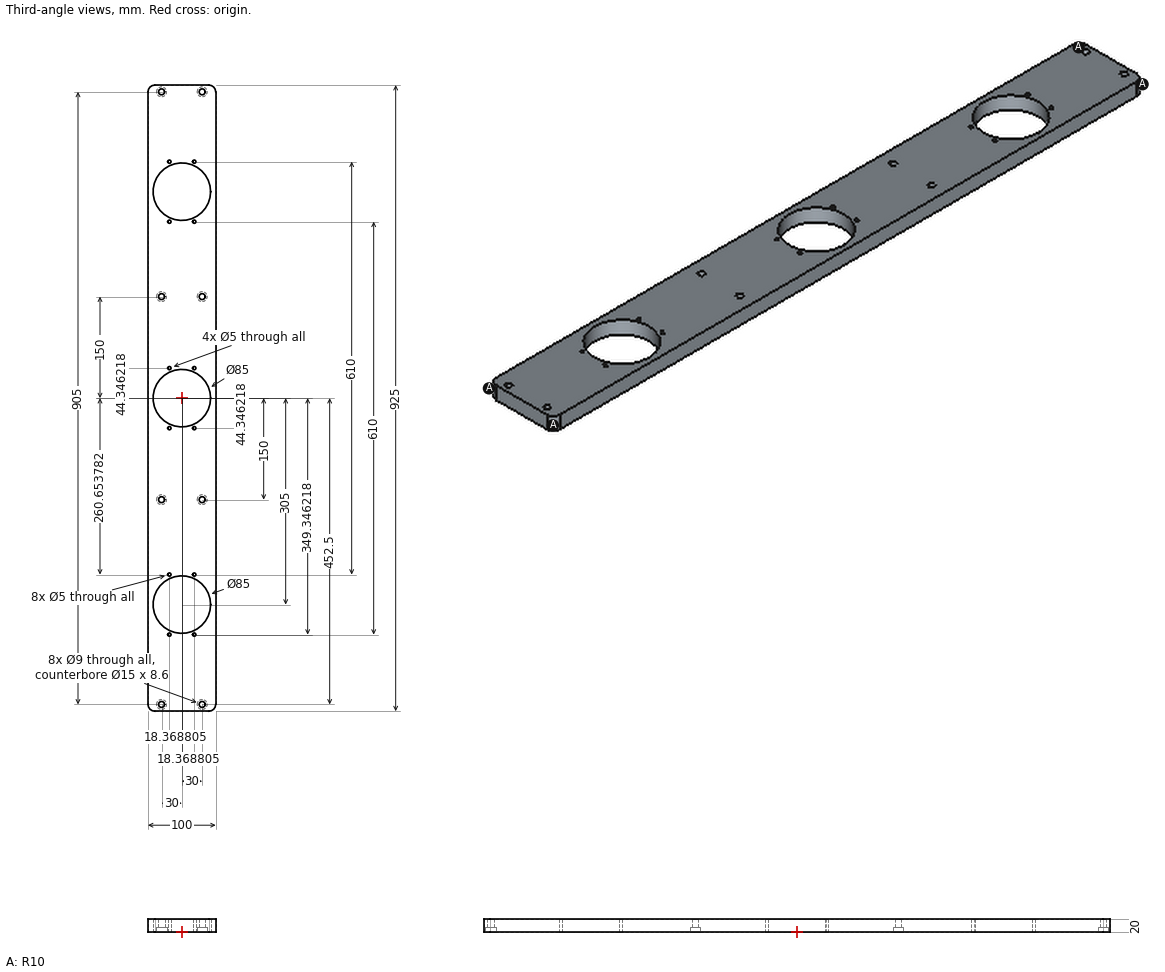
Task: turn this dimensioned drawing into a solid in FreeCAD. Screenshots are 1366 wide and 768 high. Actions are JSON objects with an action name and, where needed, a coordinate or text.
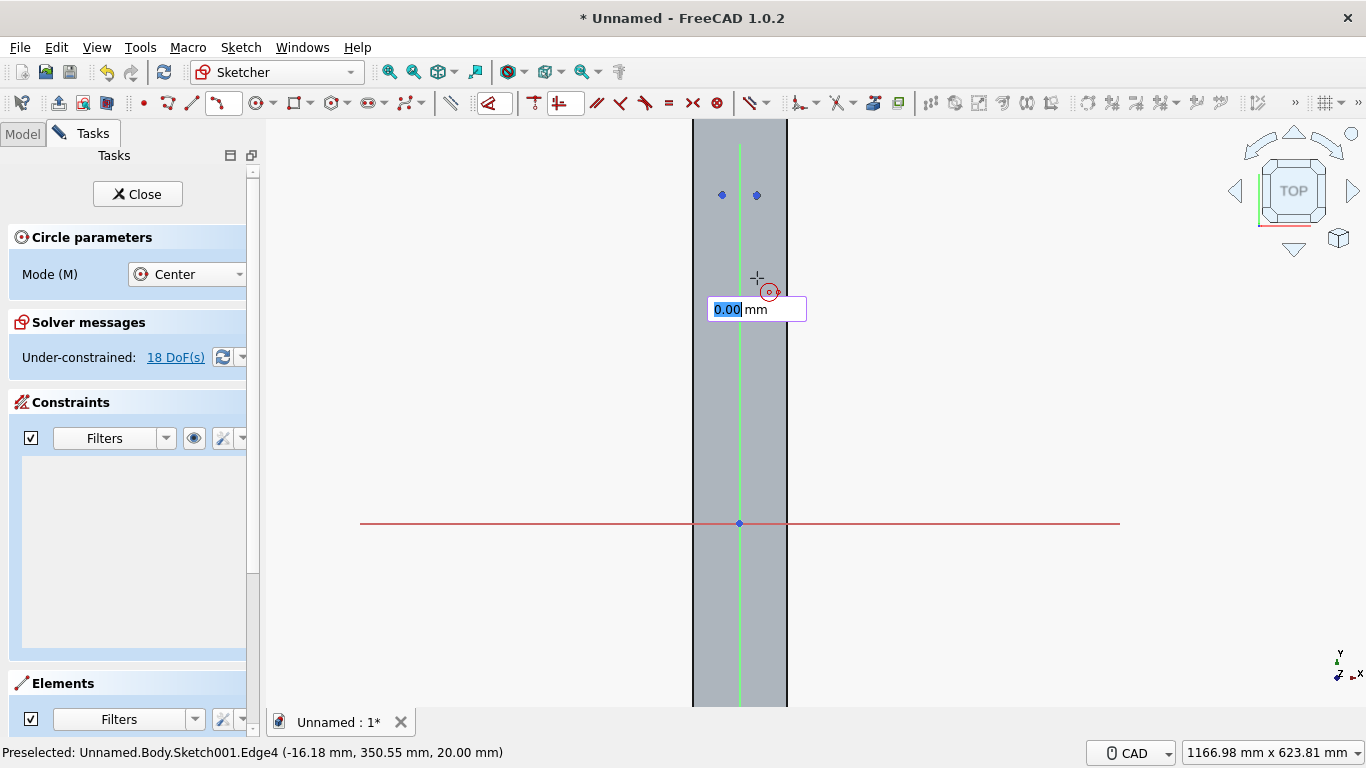
{"action": "scroll", "coordinate": [759, 277], "scroll_direction": "up", "scroll_amount": 10}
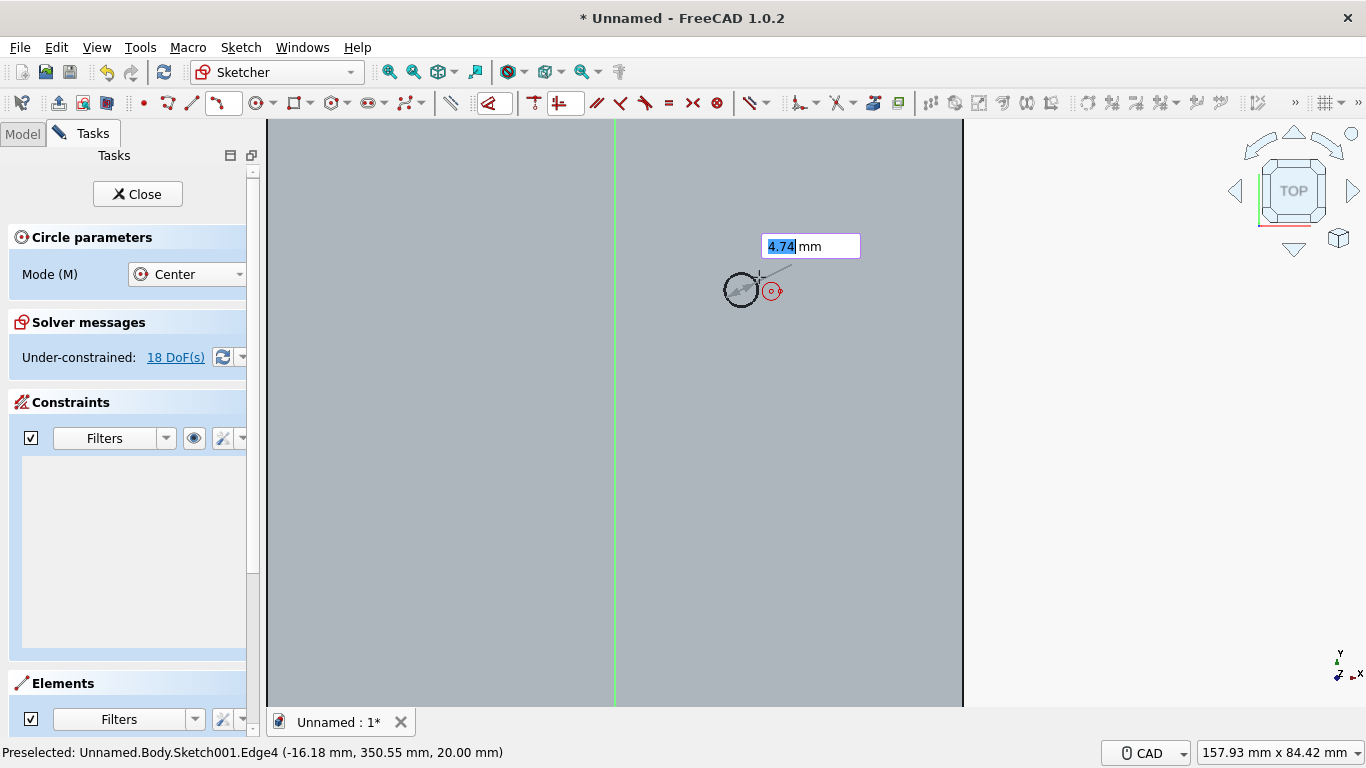
{"action": "left_click", "coordinate": [755, 272]}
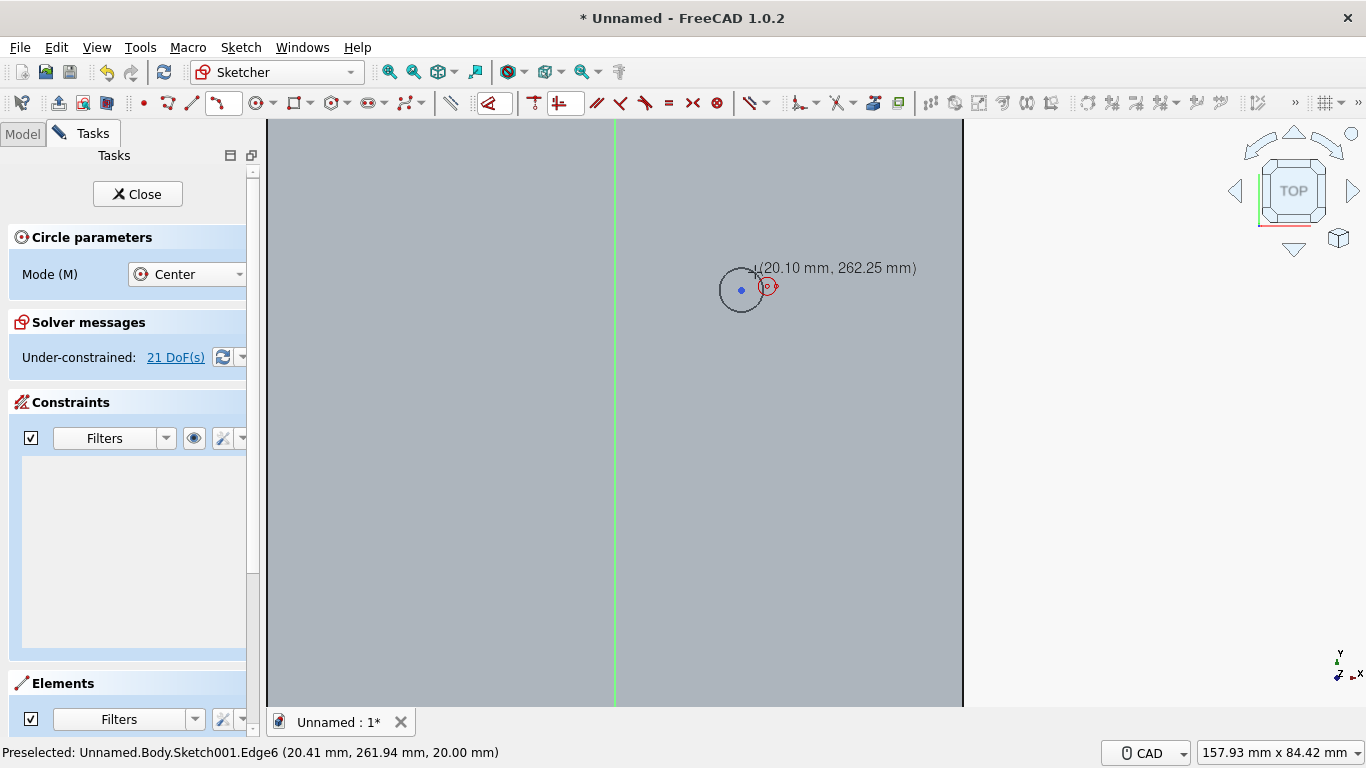
{"action": "scroll", "coordinate": [487, 284], "scroll_direction": "up", "scroll_amount": 2}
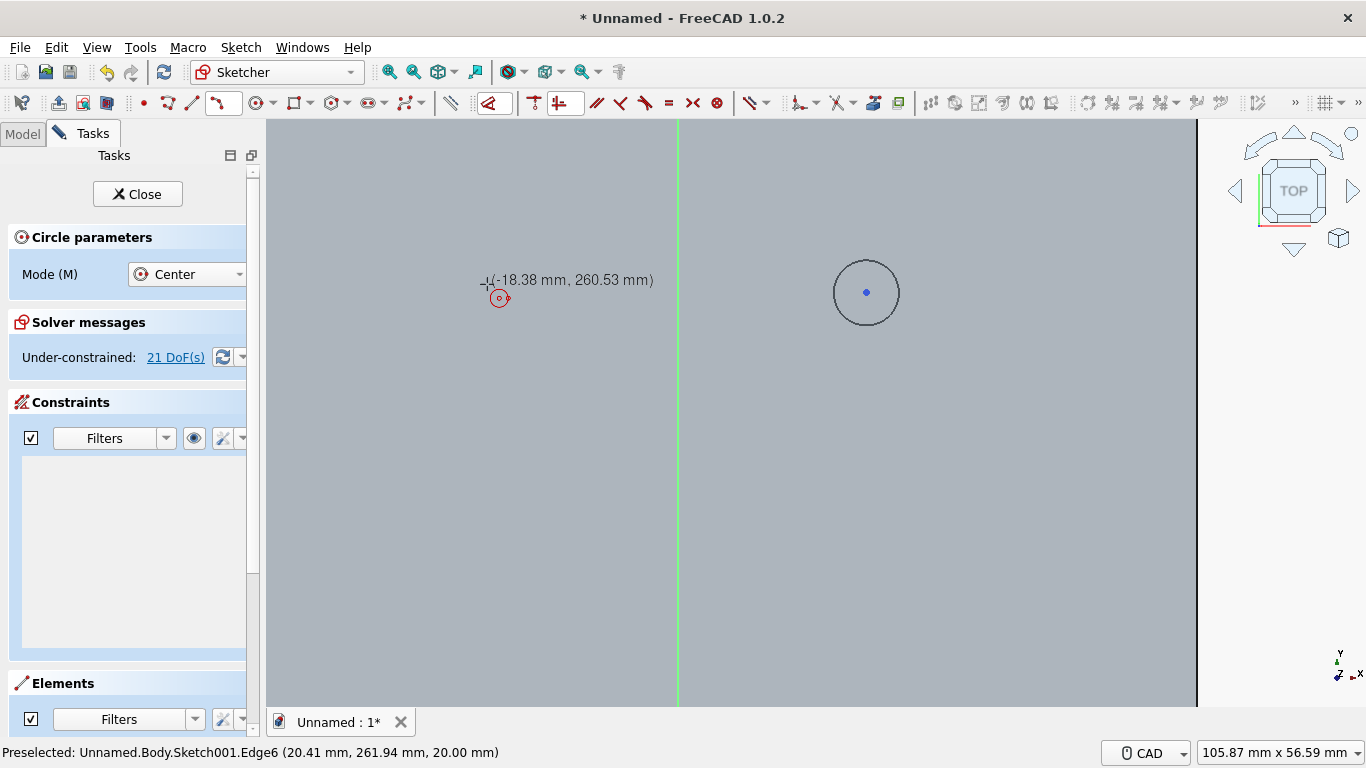
{"action": "scroll", "coordinate": [751, 278], "scroll_direction": "down", "scroll_amount": 15}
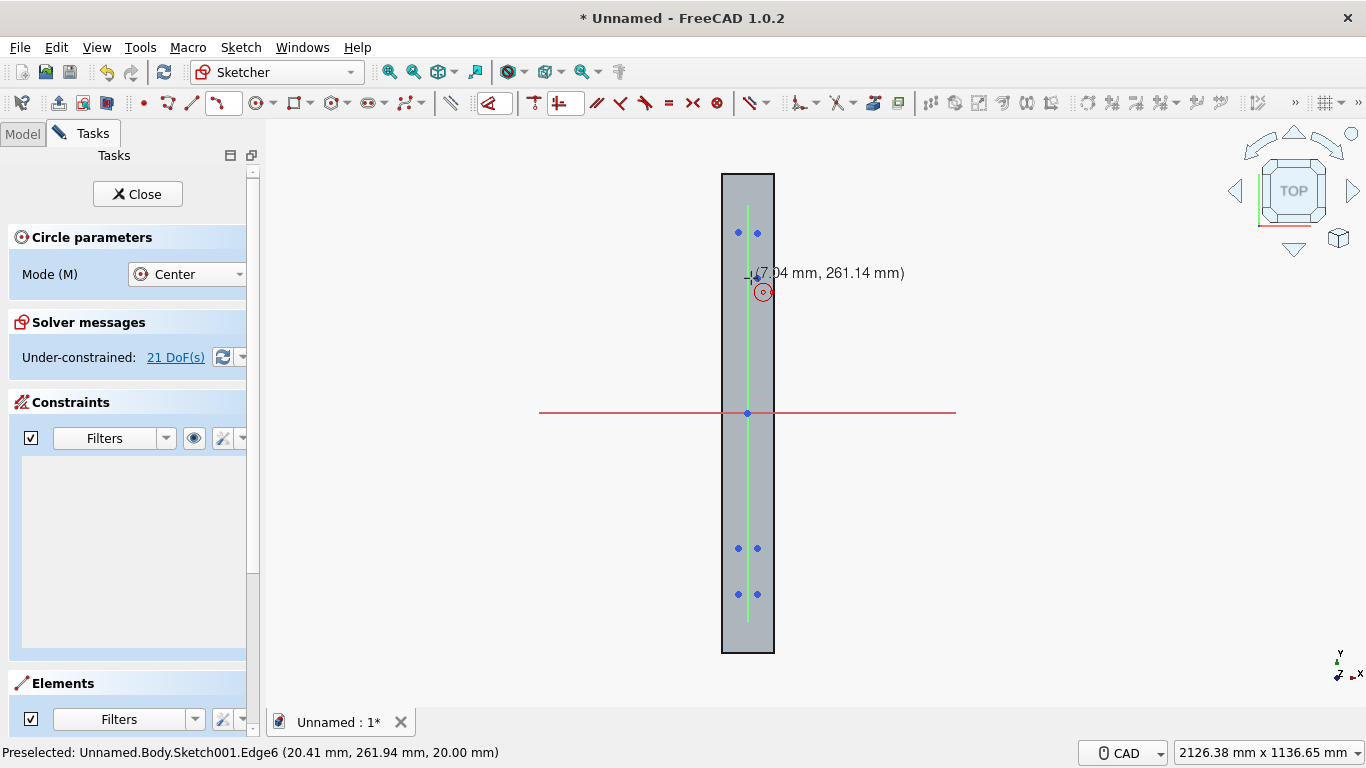
{"action": "scroll", "coordinate": [738, 279], "scroll_direction": "up", "scroll_amount": 3}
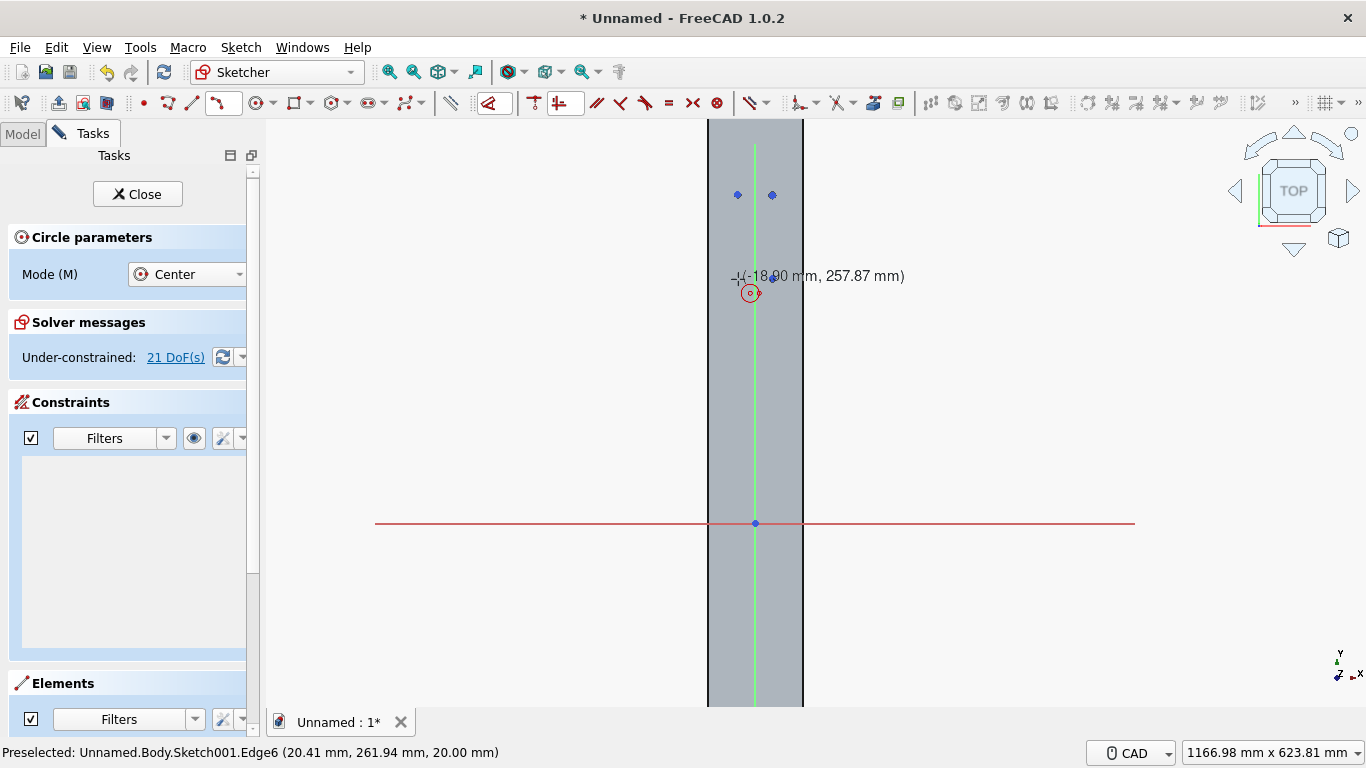
{"action": "left_click", "coordinate": [738, 278]}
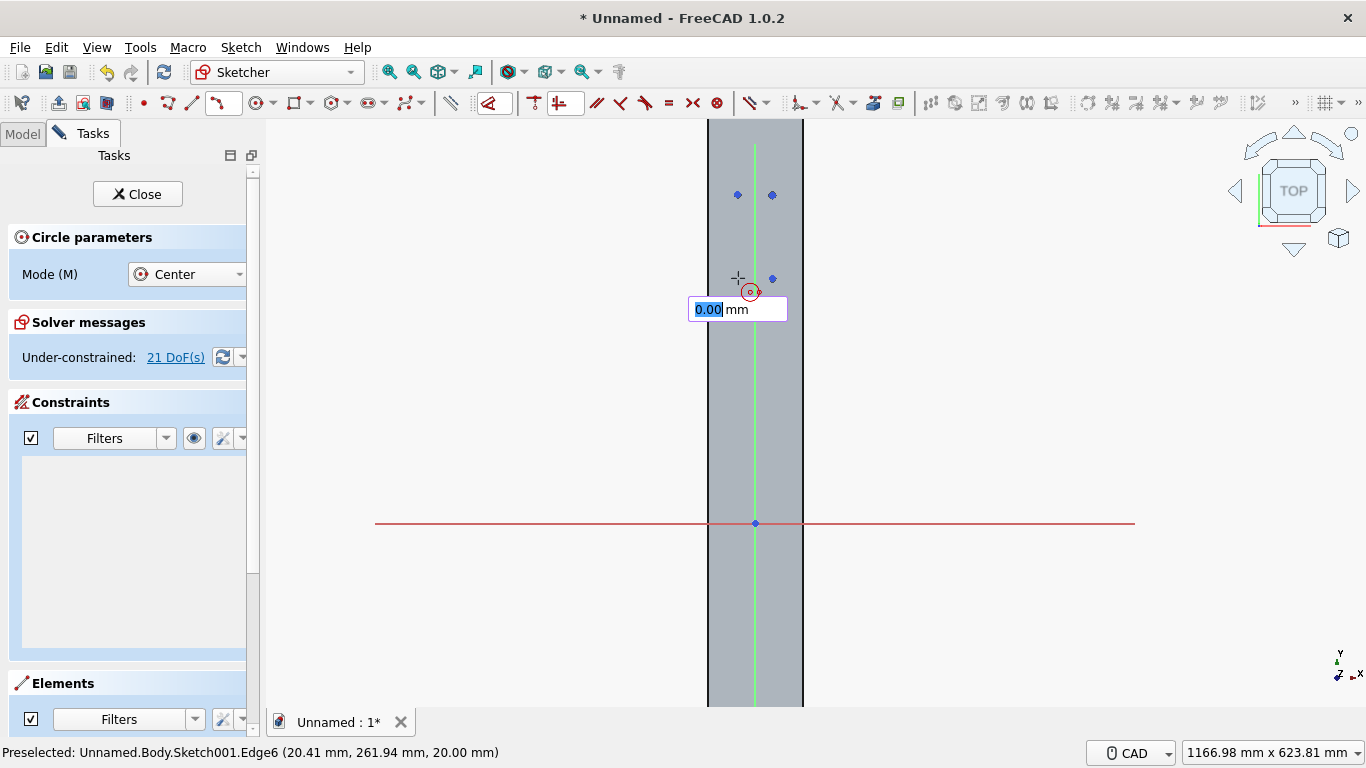
{"action": "scroll", "coordinate": [740, 276], "scroll_direction": "up", "scroll_amount": 10}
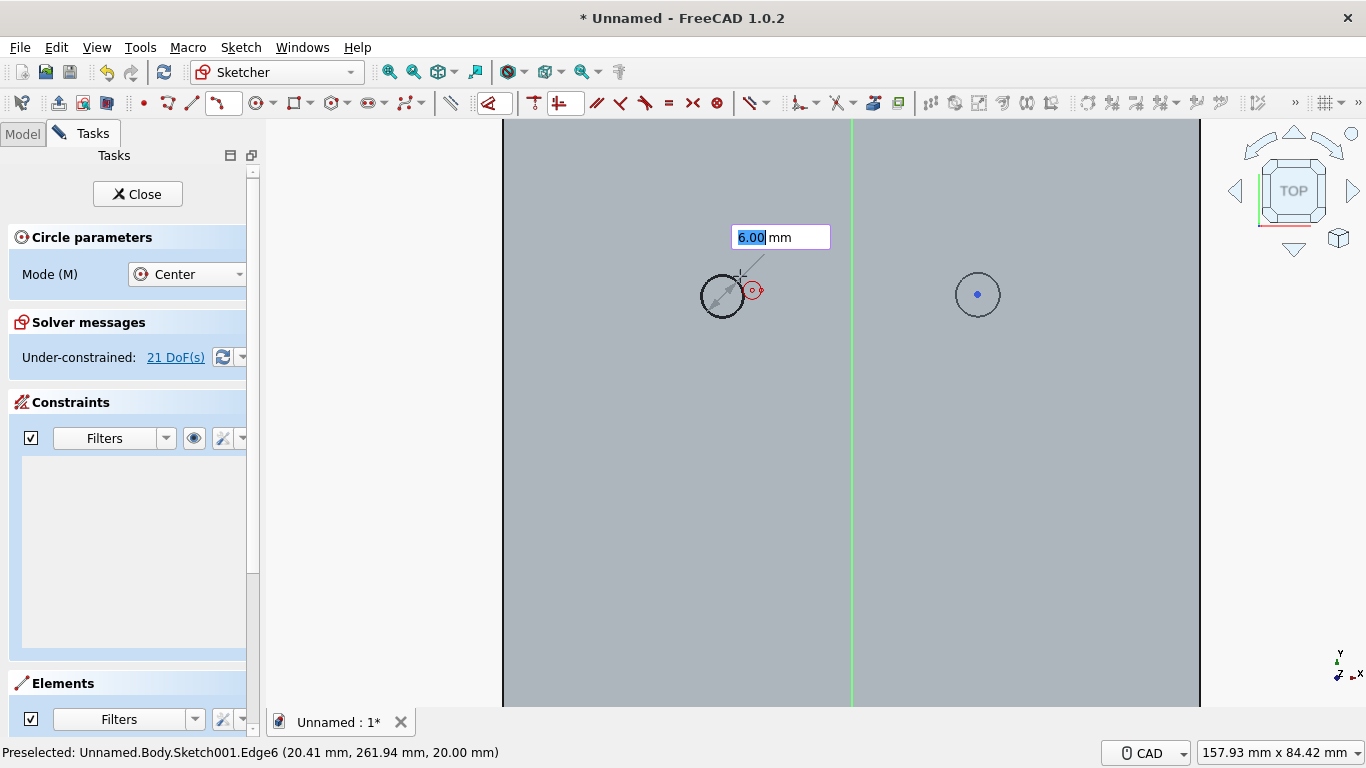
{"action": "left_click", "coordinate": [736, 277]}
{"action": "key", "text": "Escape"}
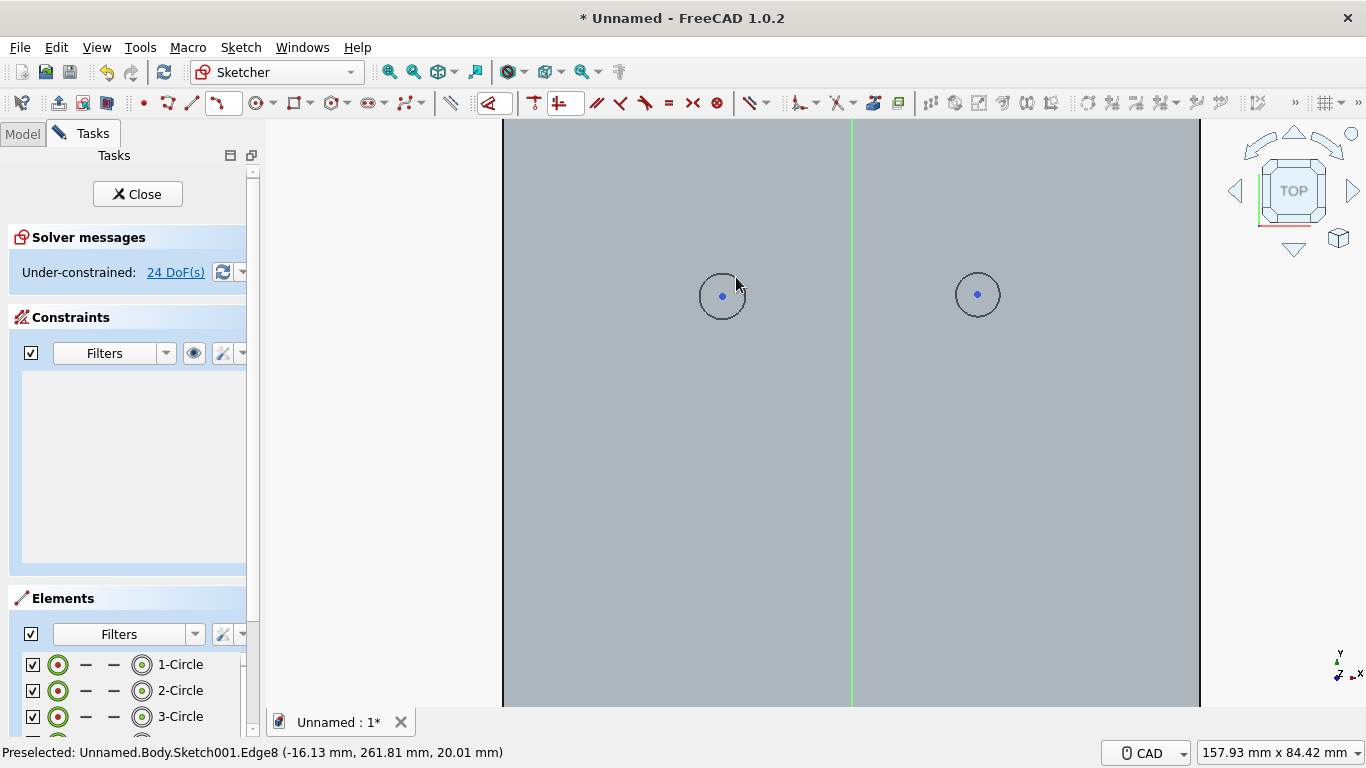
{"action": "scroll", "coordinate": [739, 277], "scroll_direction": "down", "scroll_amount": 13}